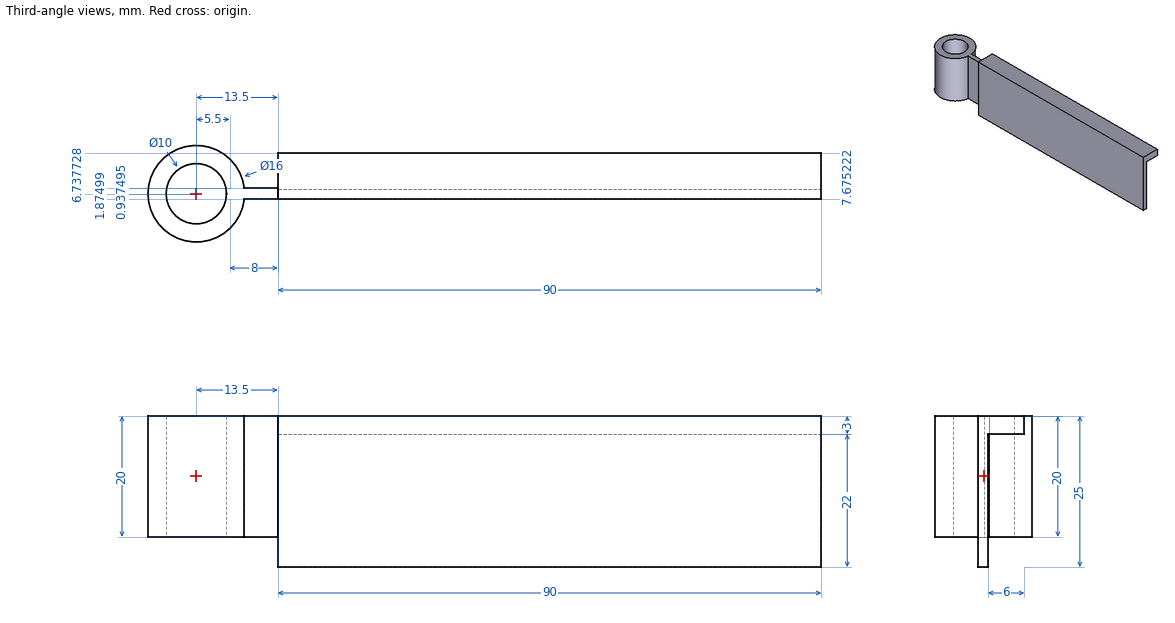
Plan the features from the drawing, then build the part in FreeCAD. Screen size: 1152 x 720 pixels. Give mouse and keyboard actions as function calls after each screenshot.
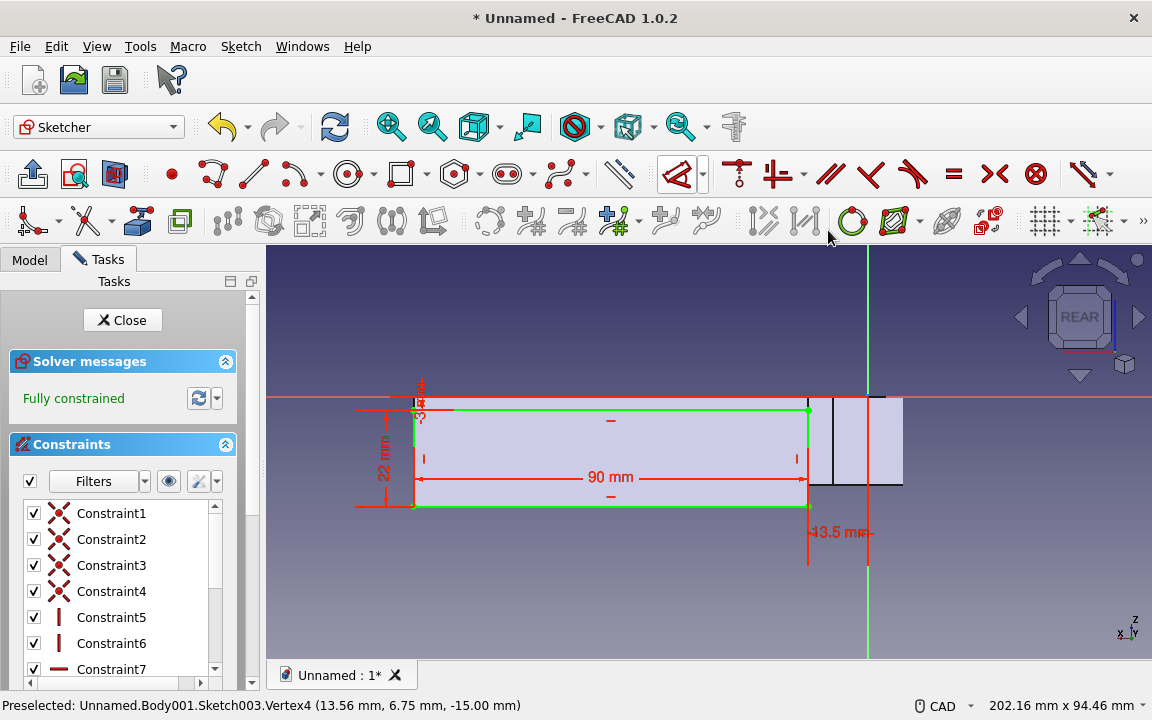
click(123, 320)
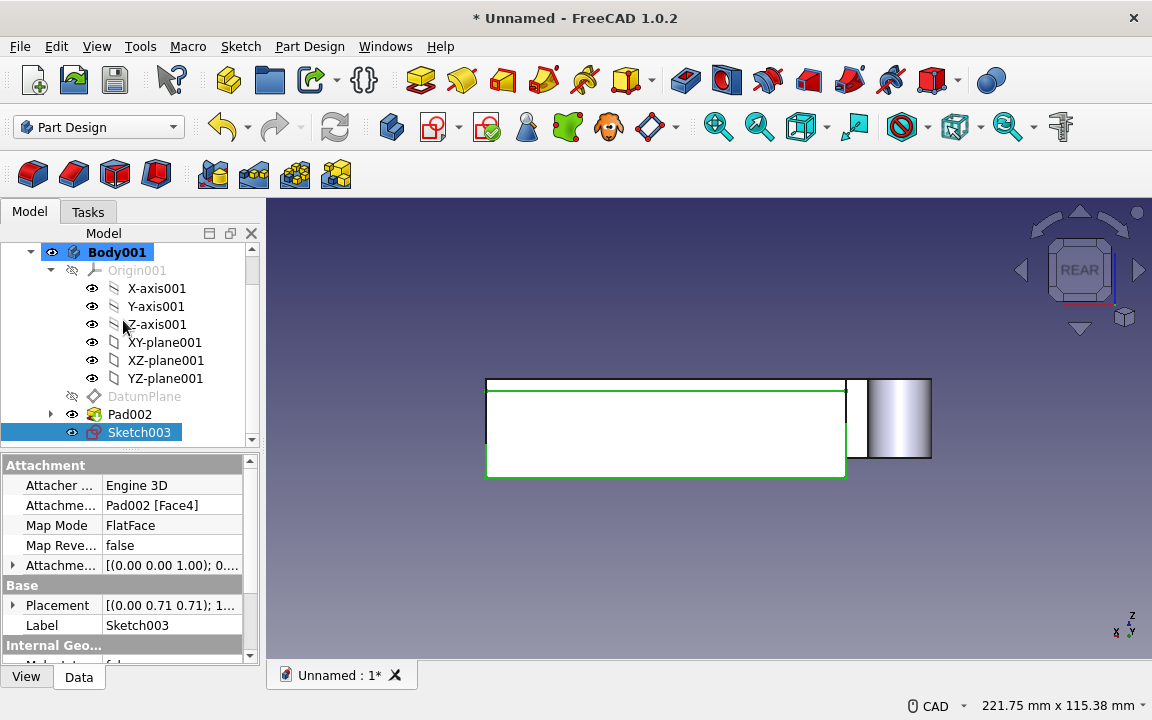
click(686, 80)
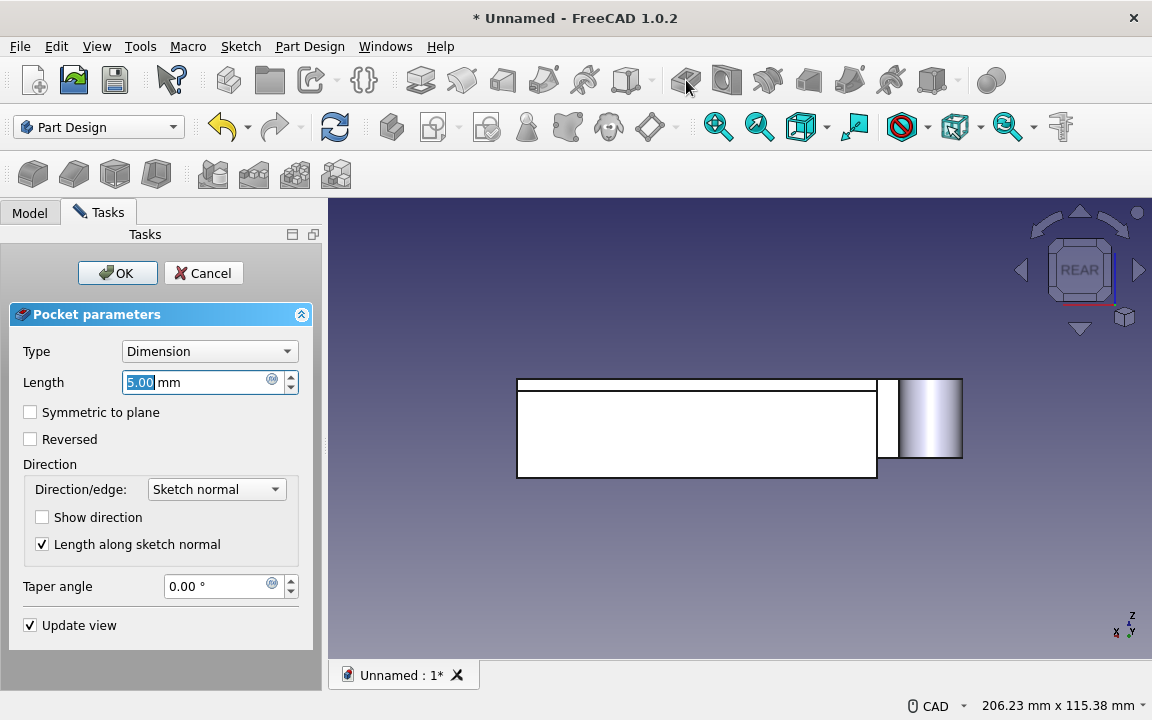
text(6)
key(Tab)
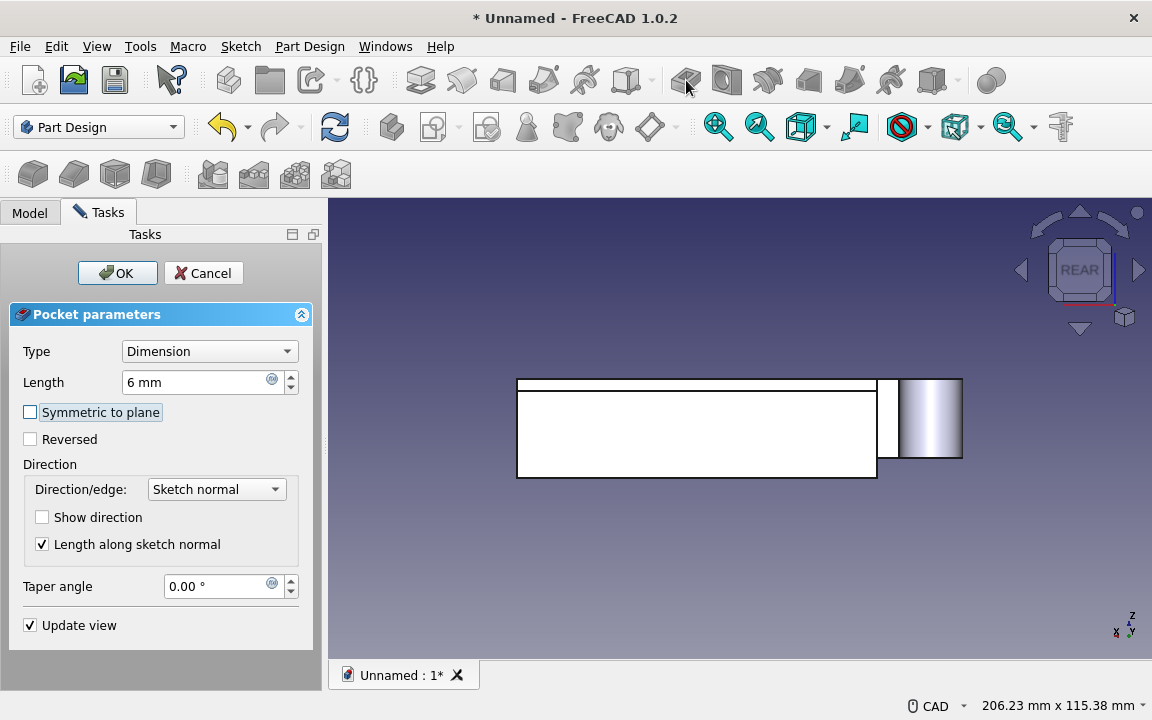
click(118, 273)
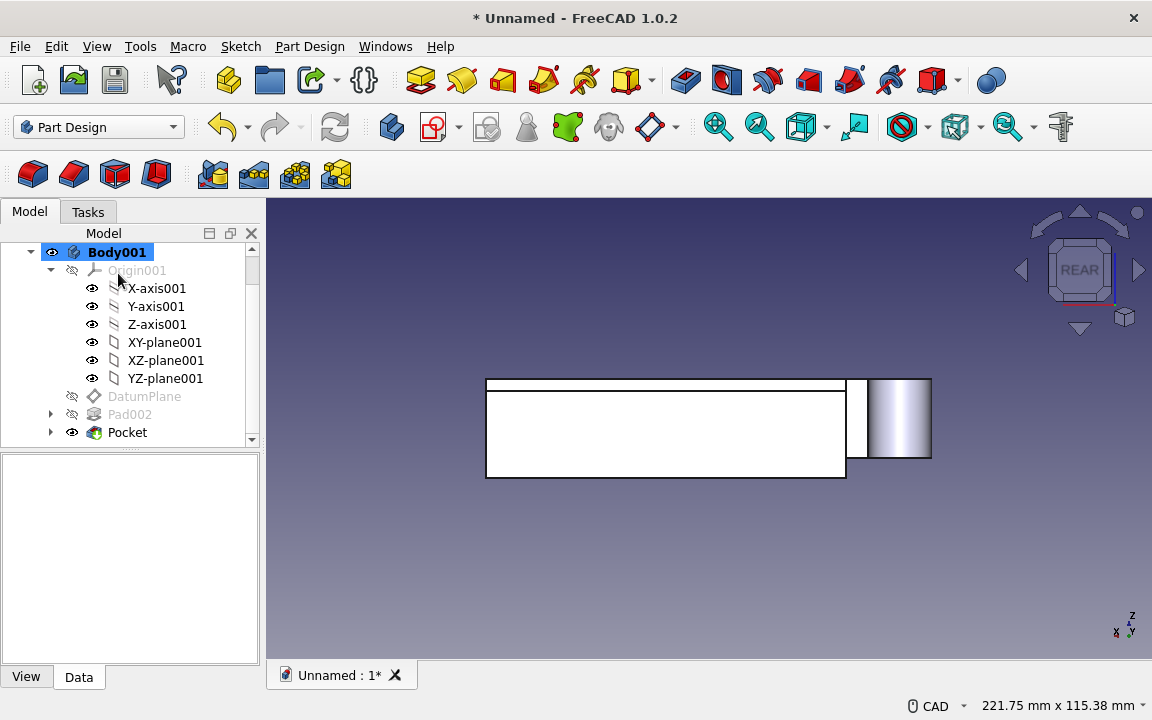
key(0)